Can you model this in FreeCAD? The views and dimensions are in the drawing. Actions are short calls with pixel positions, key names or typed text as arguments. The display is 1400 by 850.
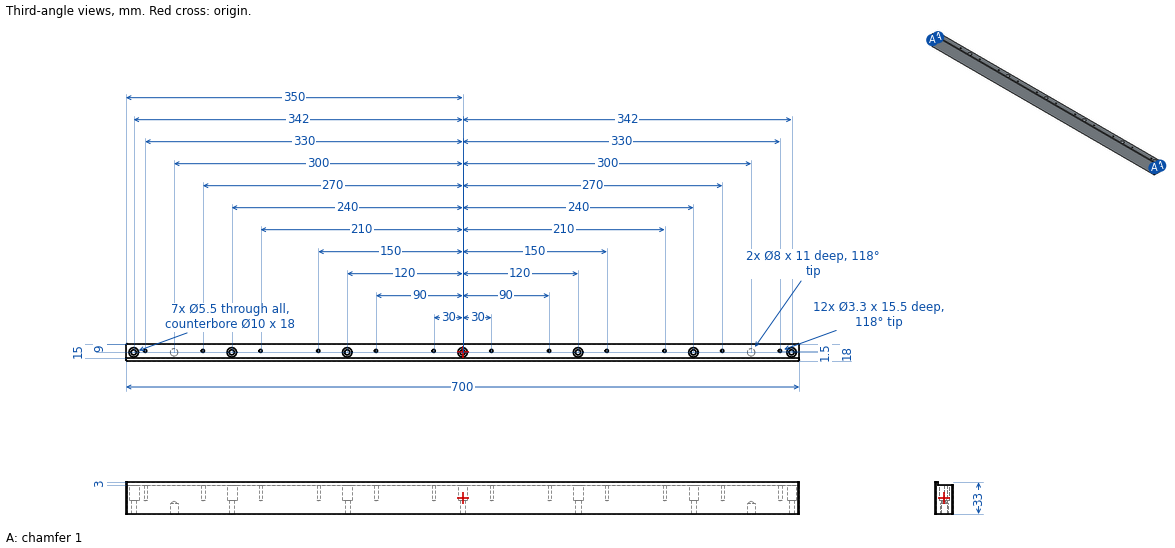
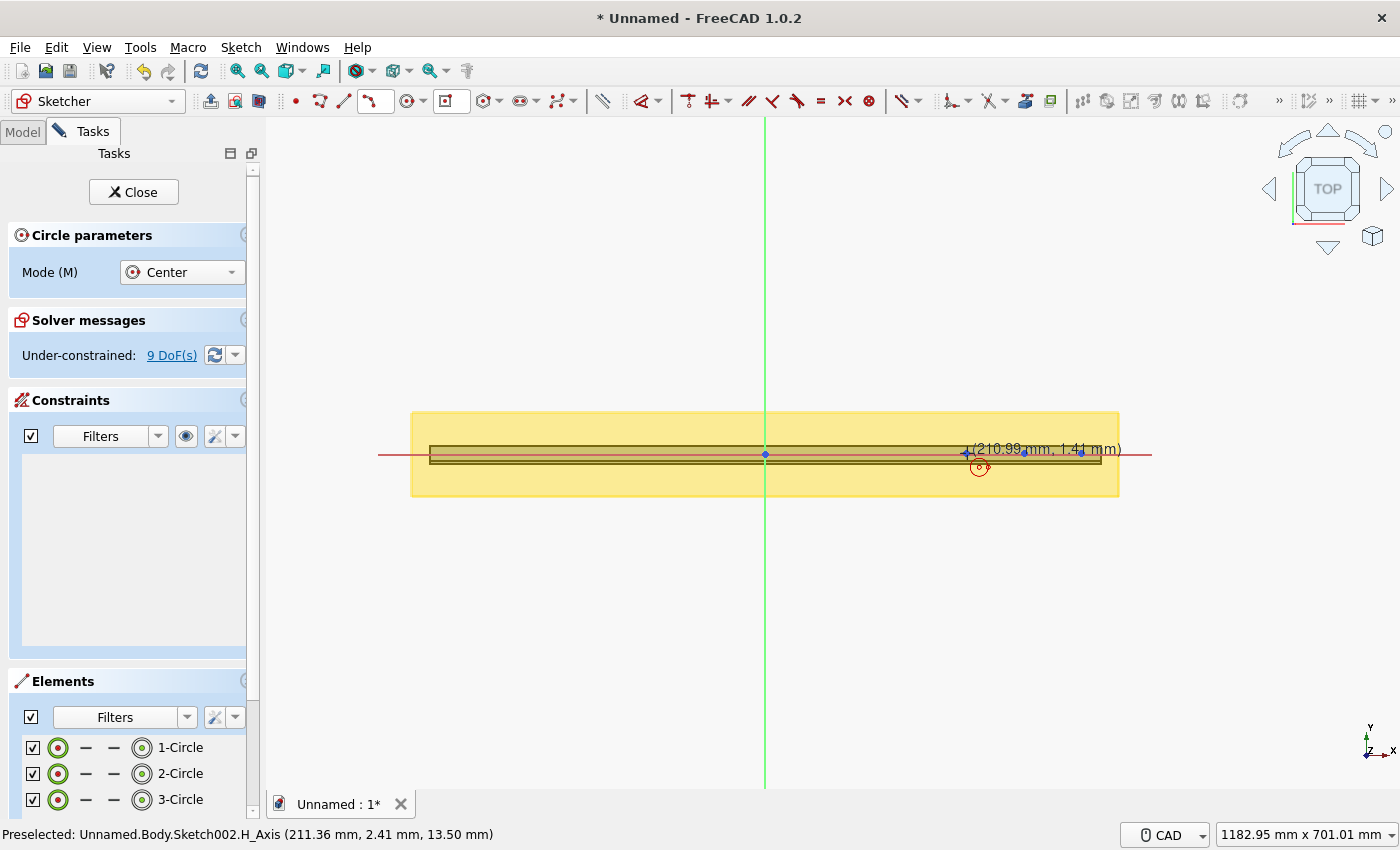
scroll(909, 453, up, 14)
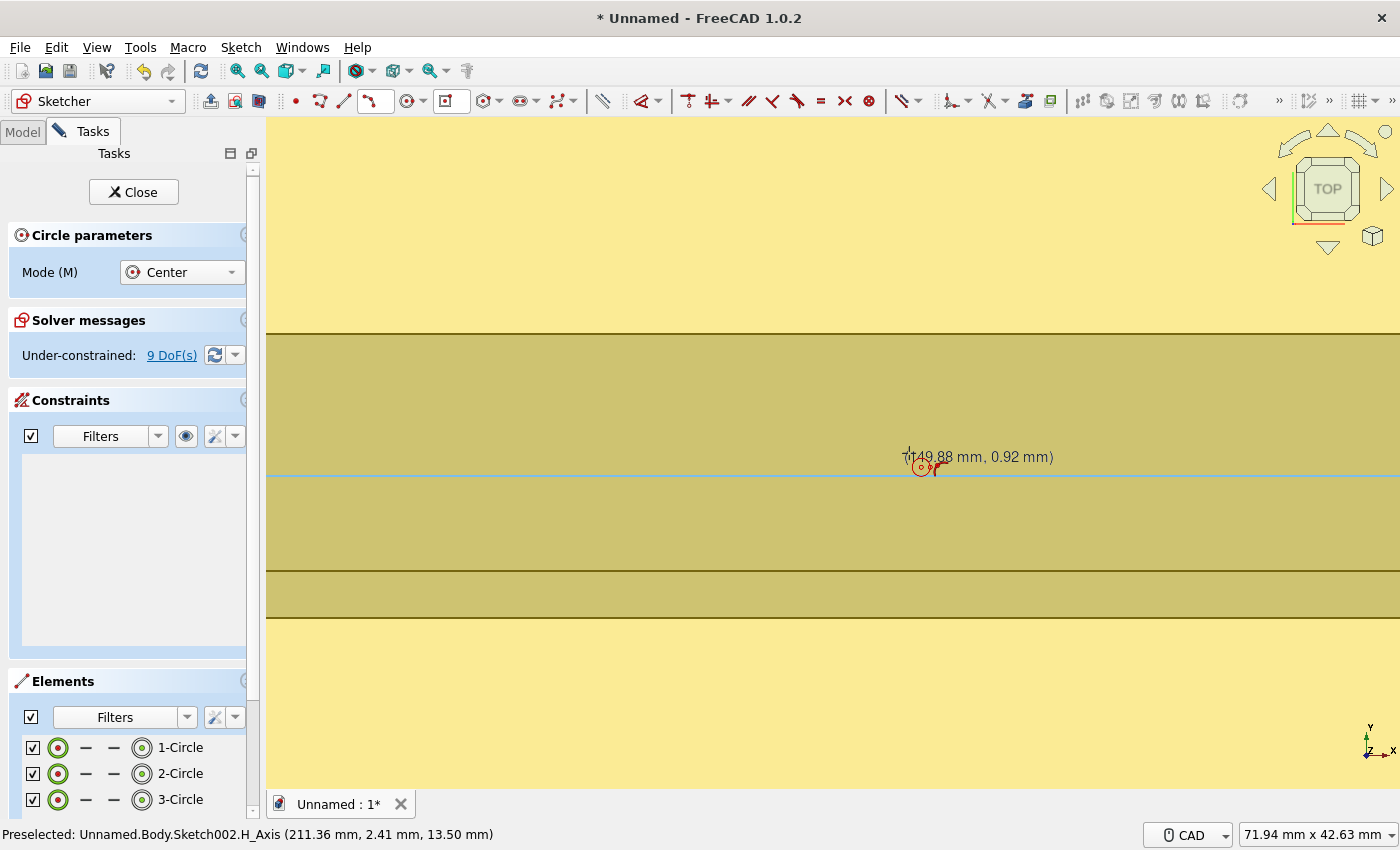
click(902, 453)
click(920, 434)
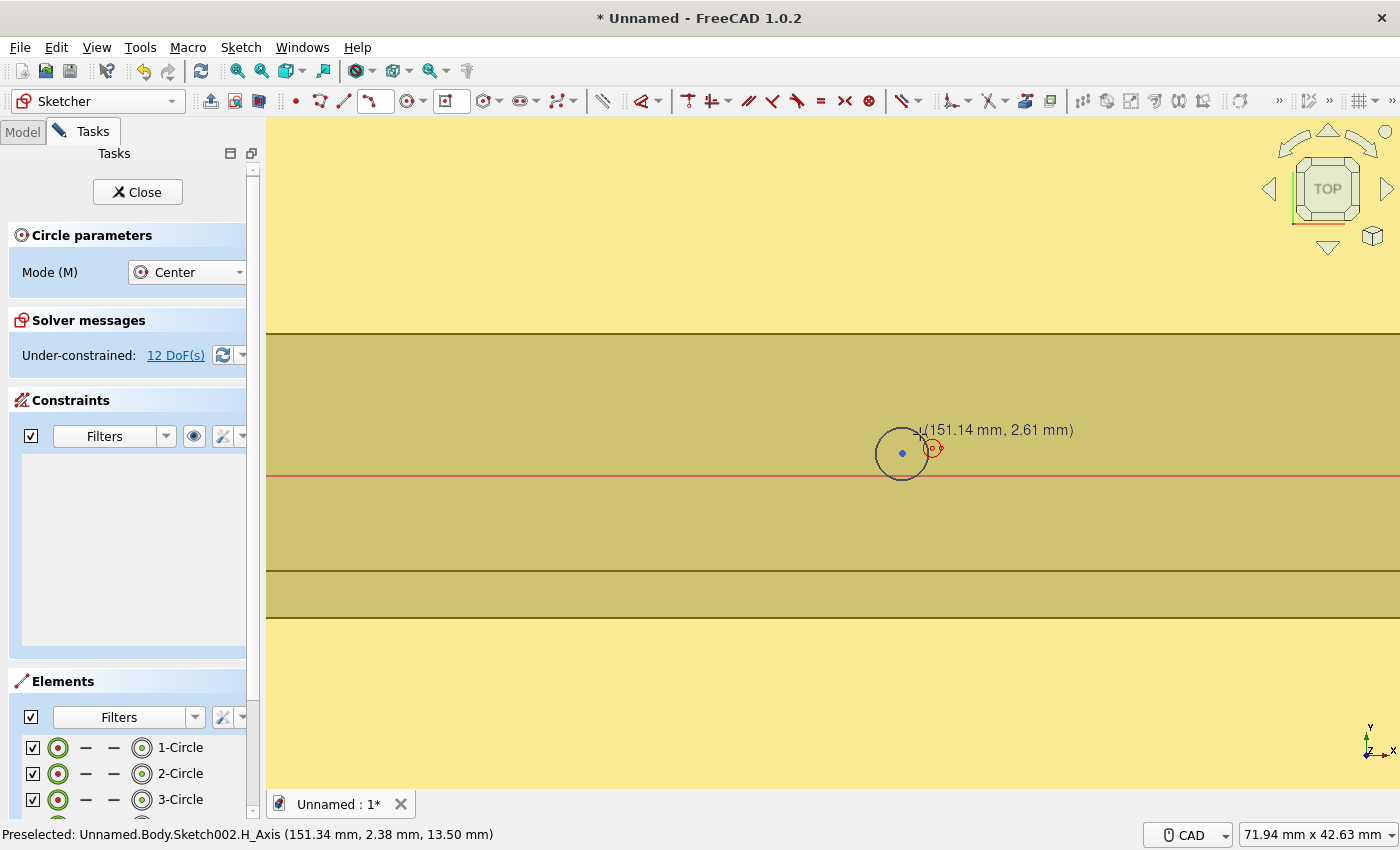
scroll(909, 453, down, 14)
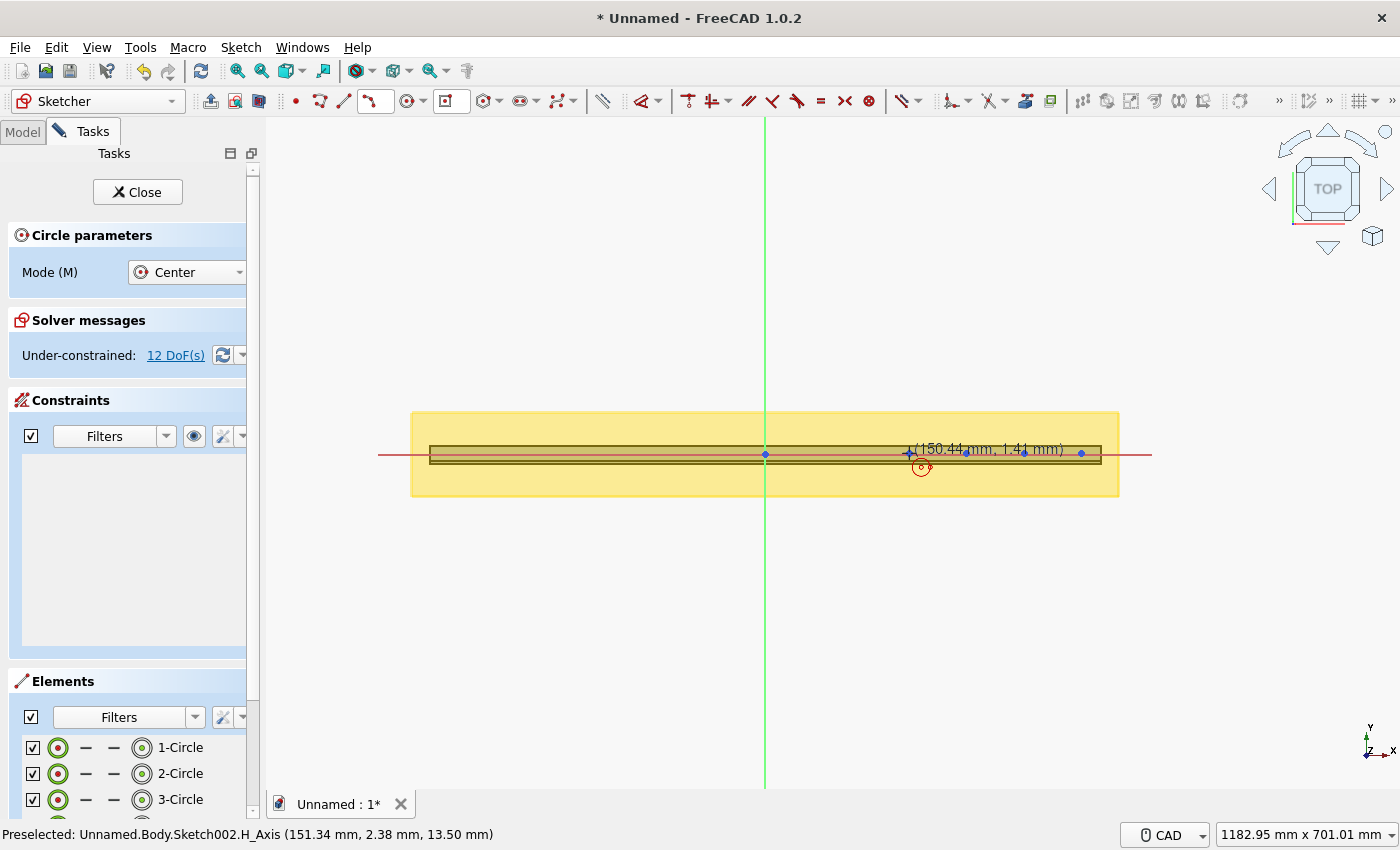
scroll(852, 453, up, 14)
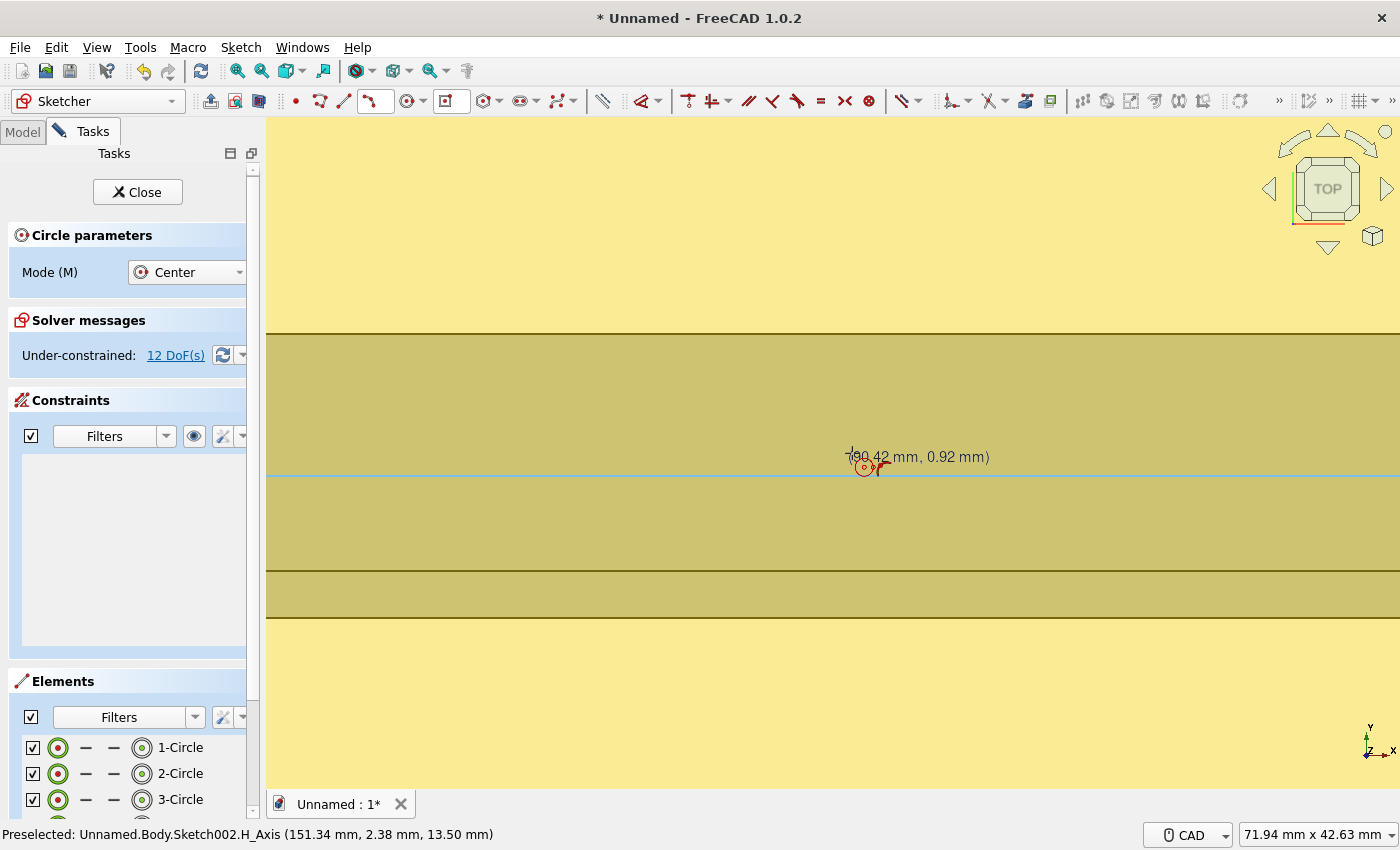
click(837, 453)
click(856, 434)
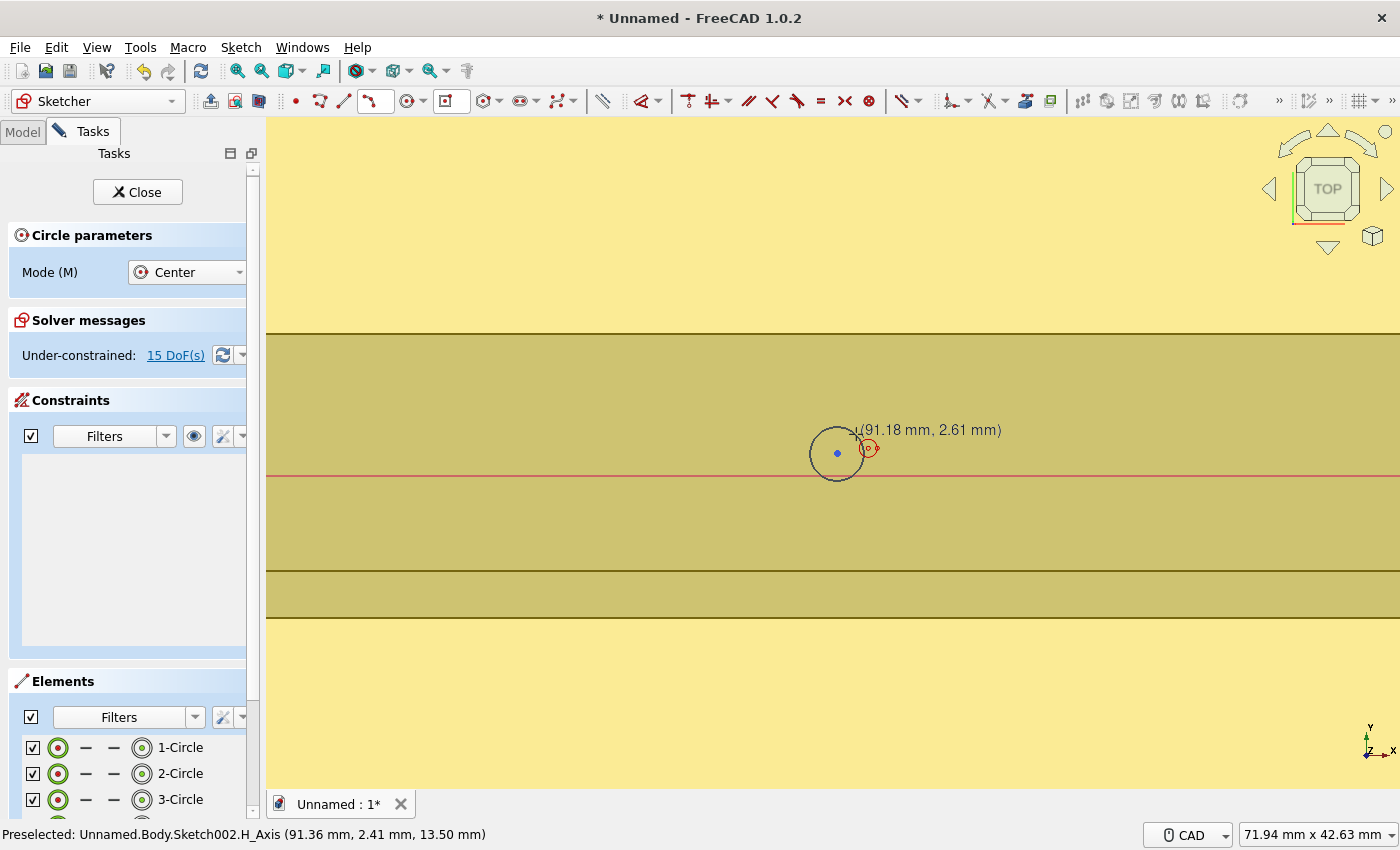
scroll(852, 453, down, 14)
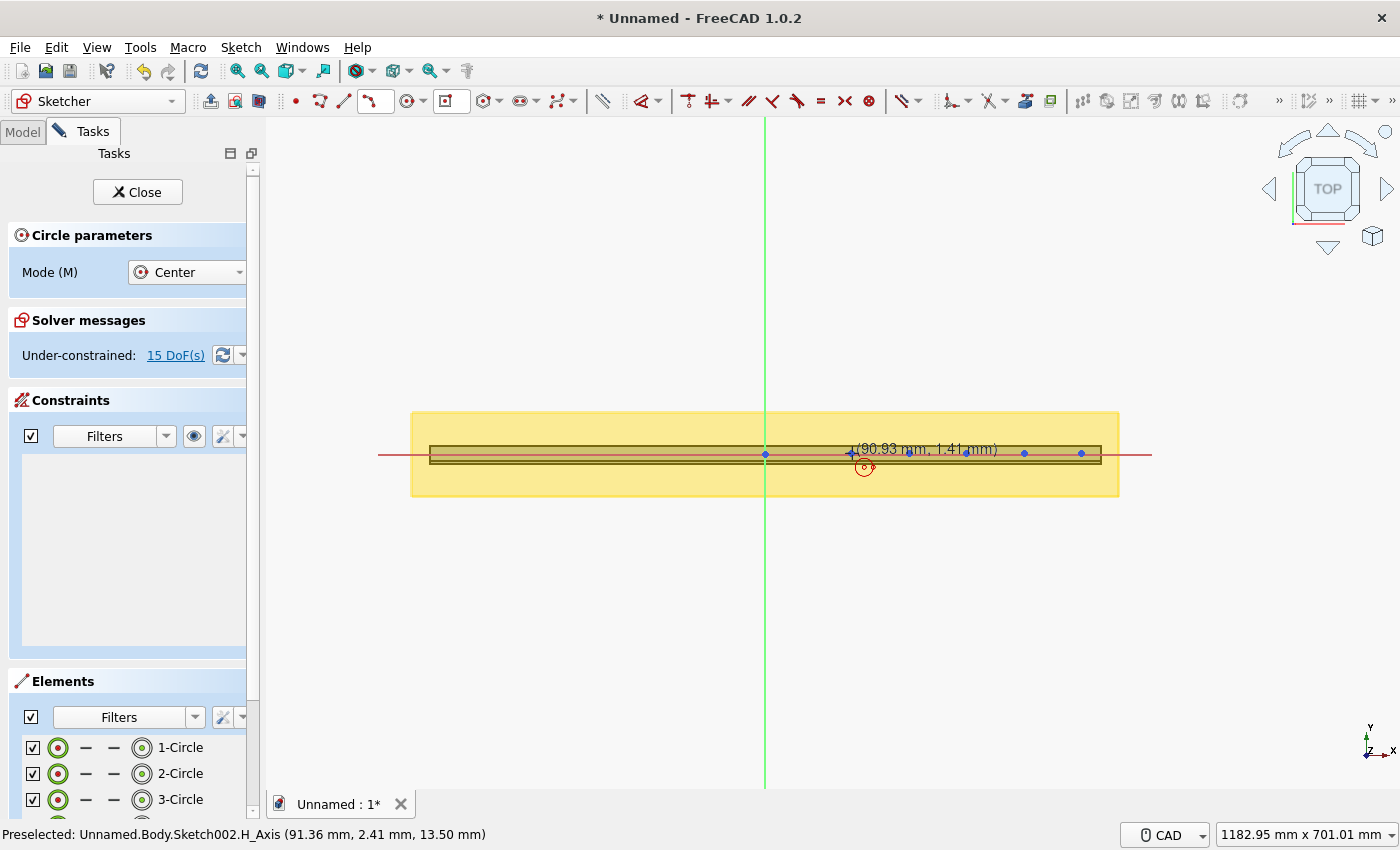
scroll(794, 453, up, 14)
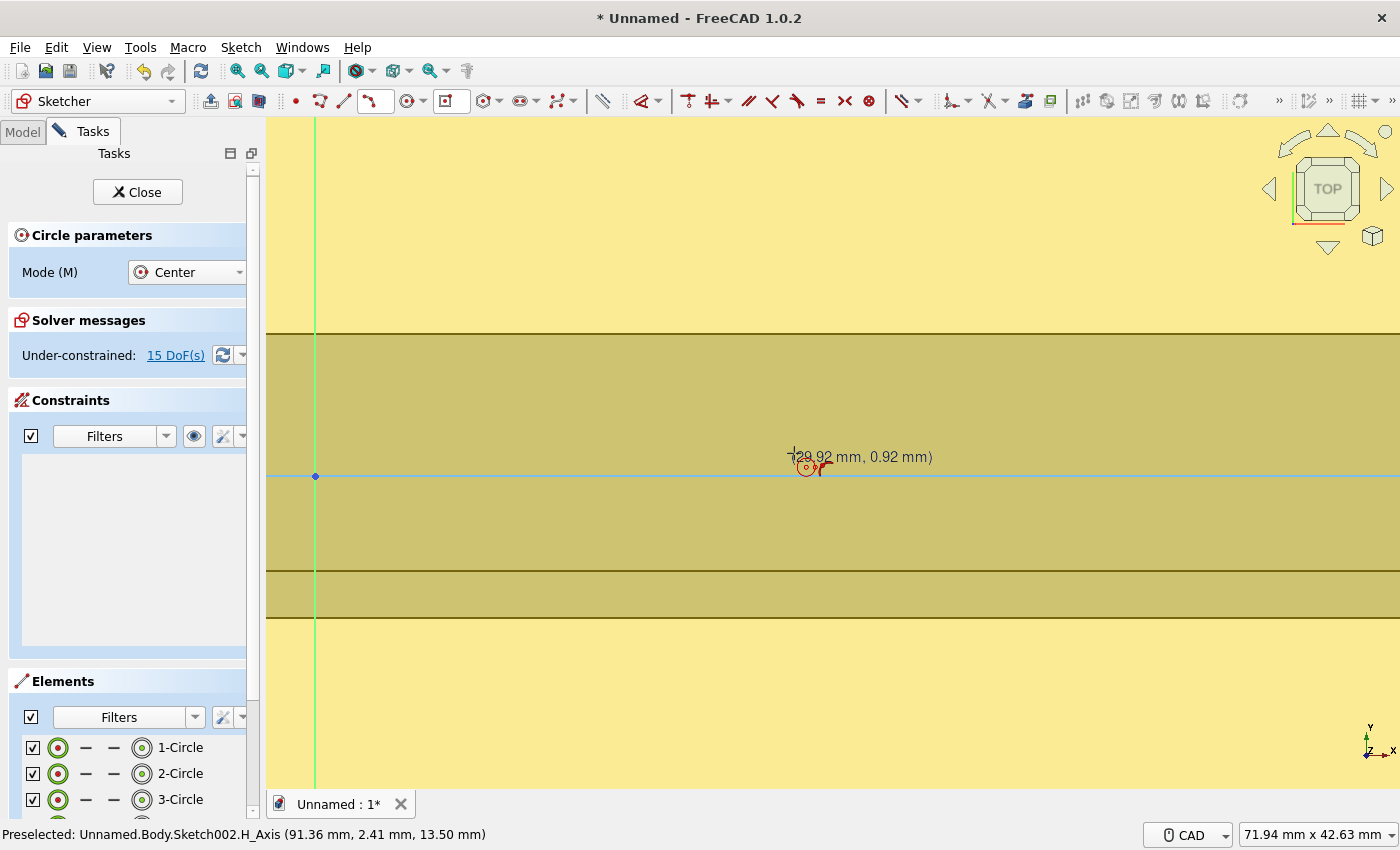
click(788, 453)
click(806, 434)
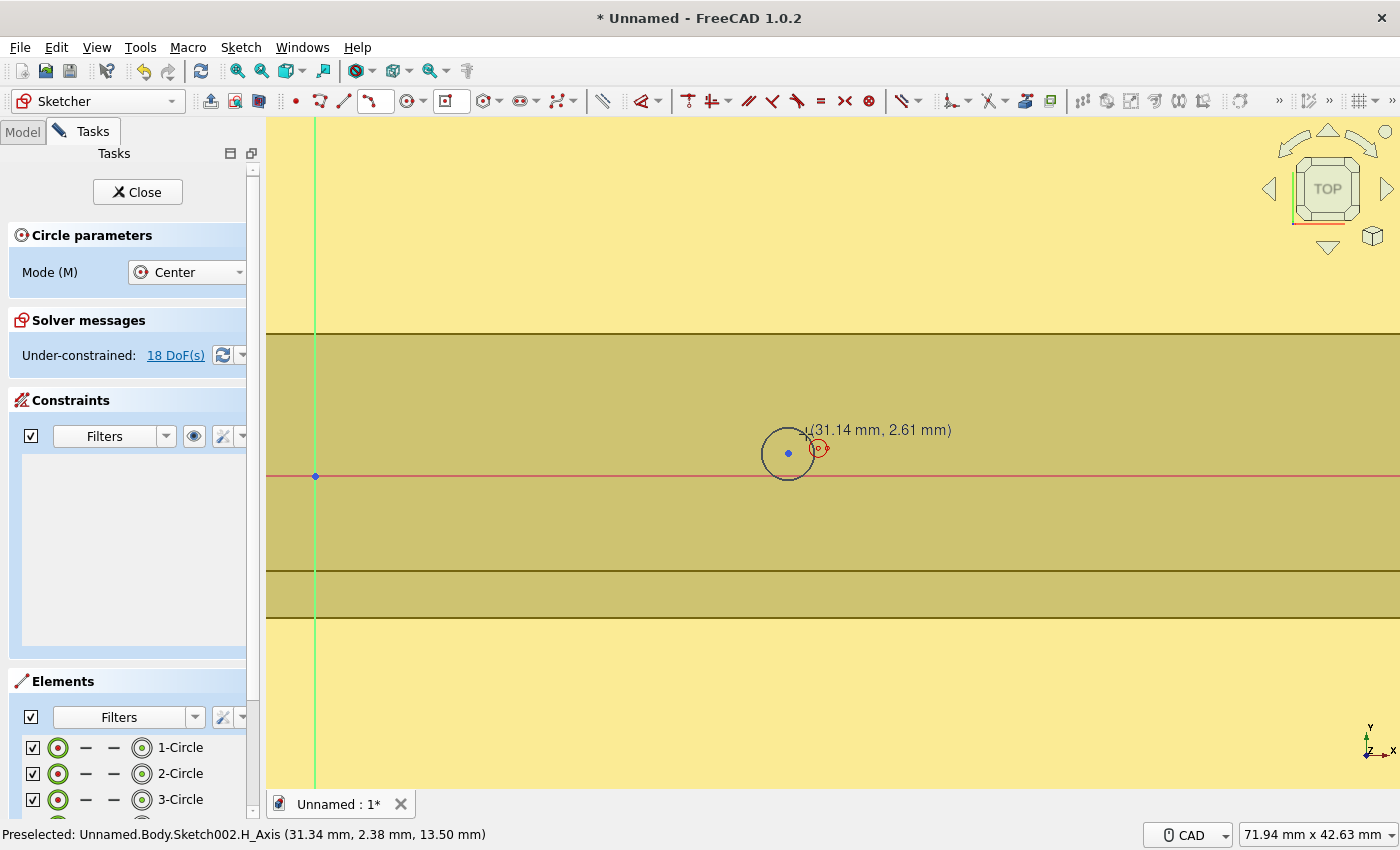
scroll(794, 453, down, 14)